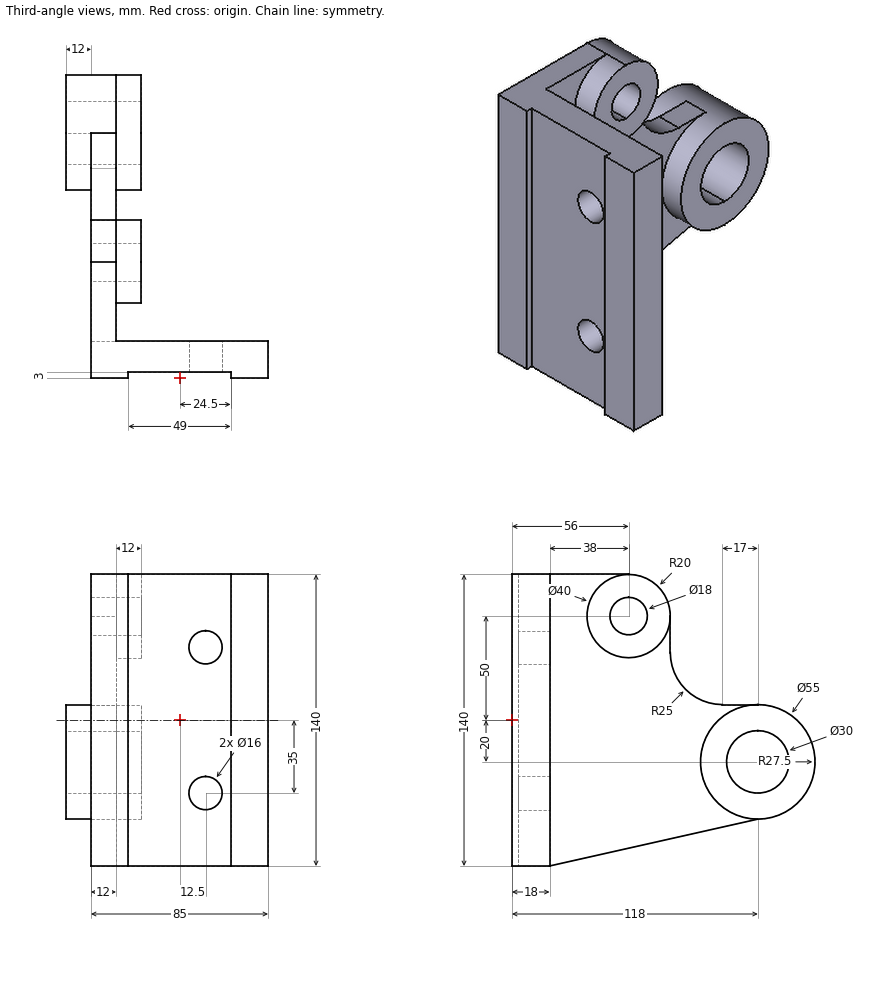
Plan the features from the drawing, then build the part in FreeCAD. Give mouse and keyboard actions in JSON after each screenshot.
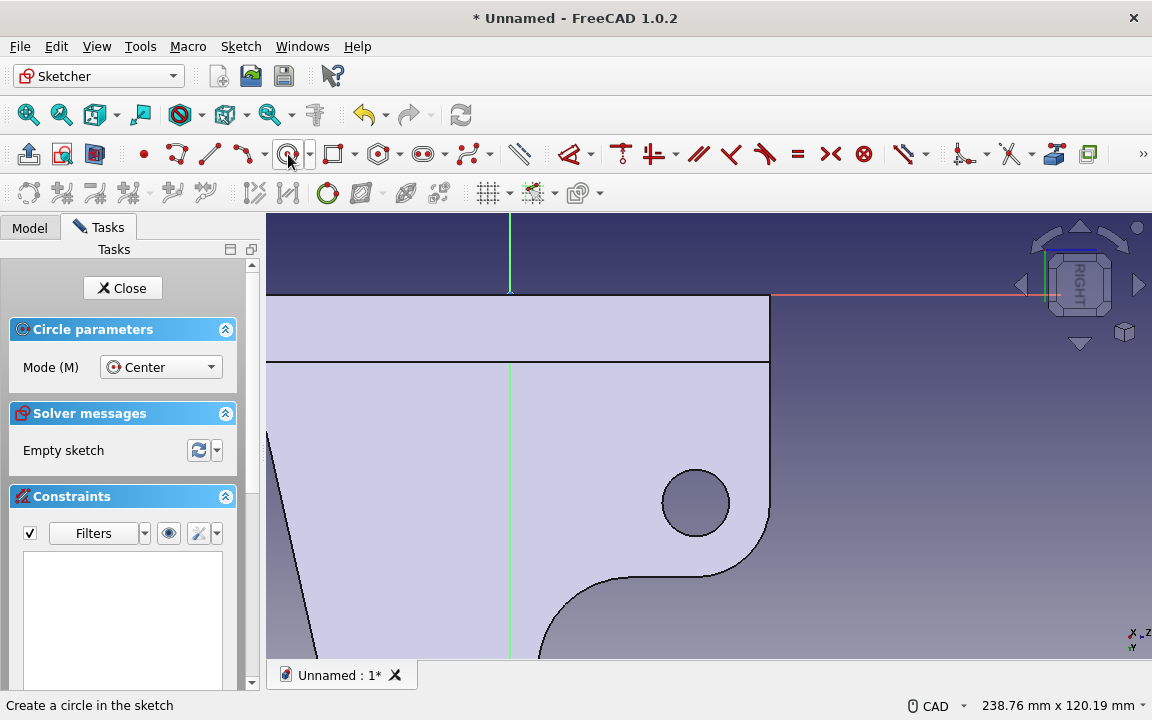
{"action": "left_click", "coordinate": [696, 503]}
{"action": "mouse_move", "coordinate": [748, 451]}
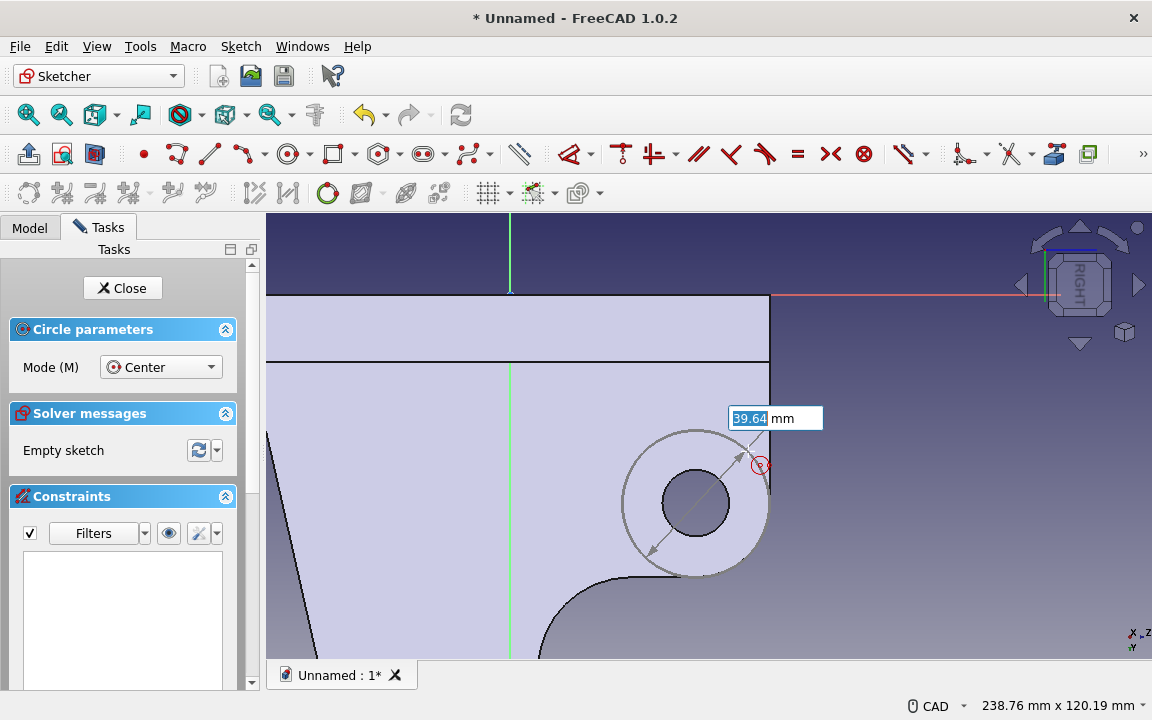
{"action": "type", "text": "40"}
{"action": "key", "text": "Return"}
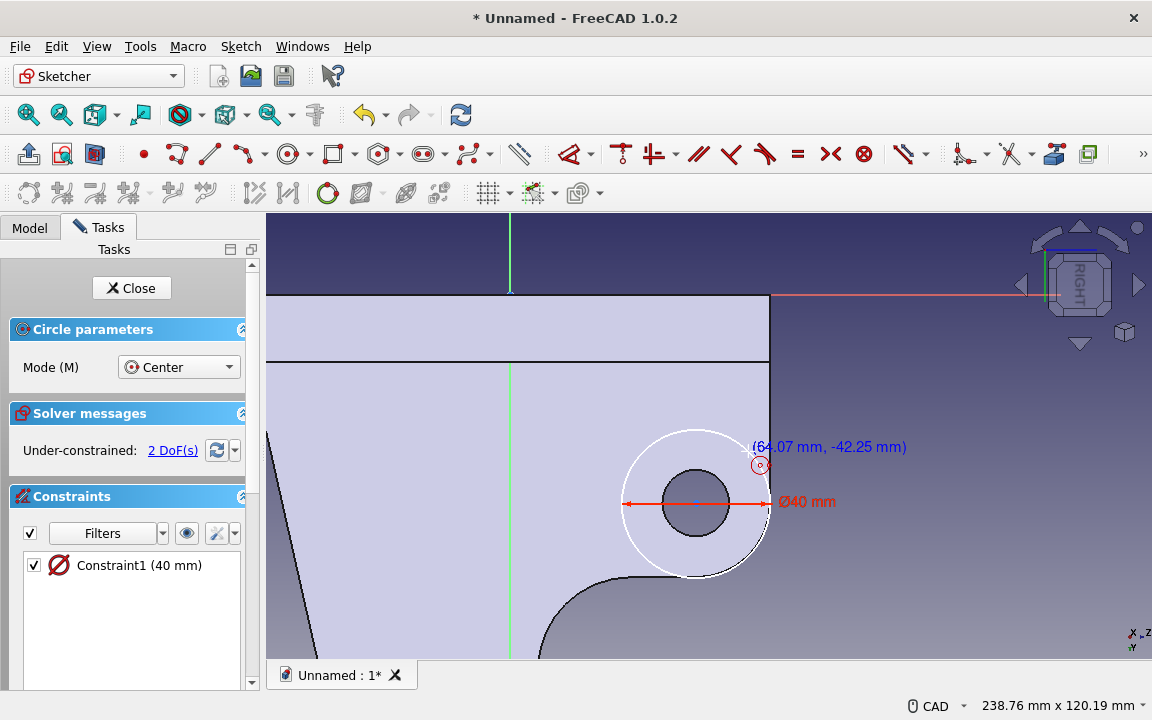
{"action": "left_click", "coordinate": [696, 504]}
{"action": "mouse_move", "coordinate": [719, 479]}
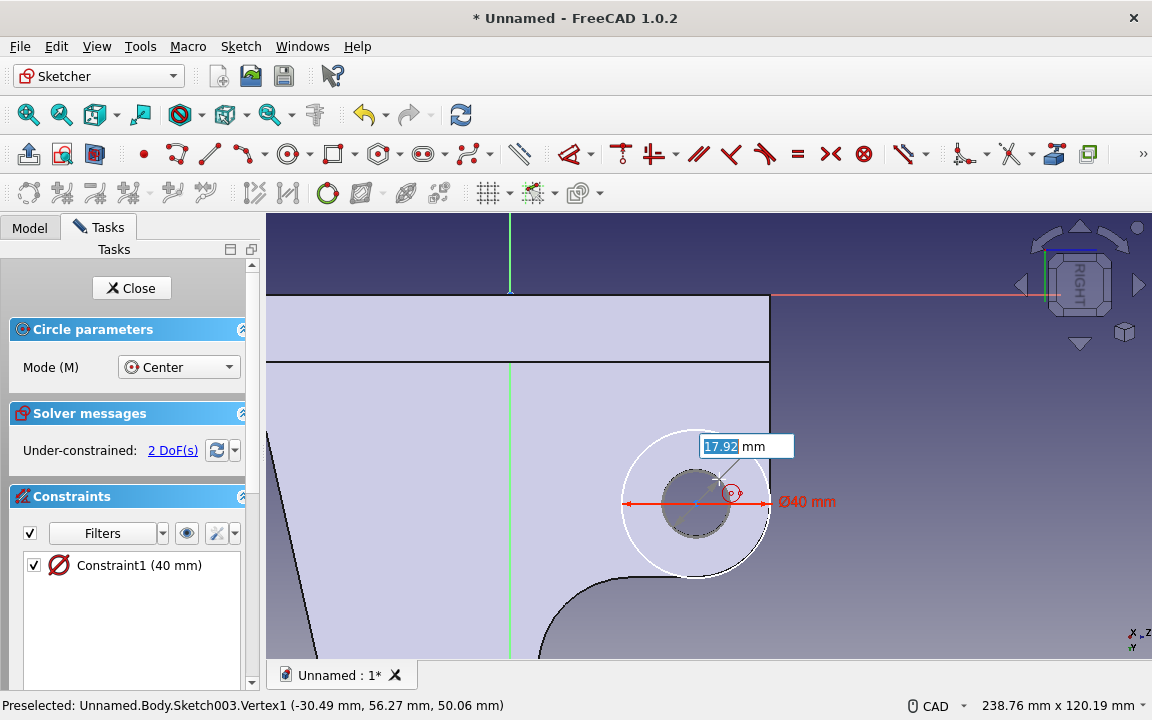
{"action": "type", "text": "18"}
{"action": "key", "text": "Return"}
{"action": "key", "text": "Escape"}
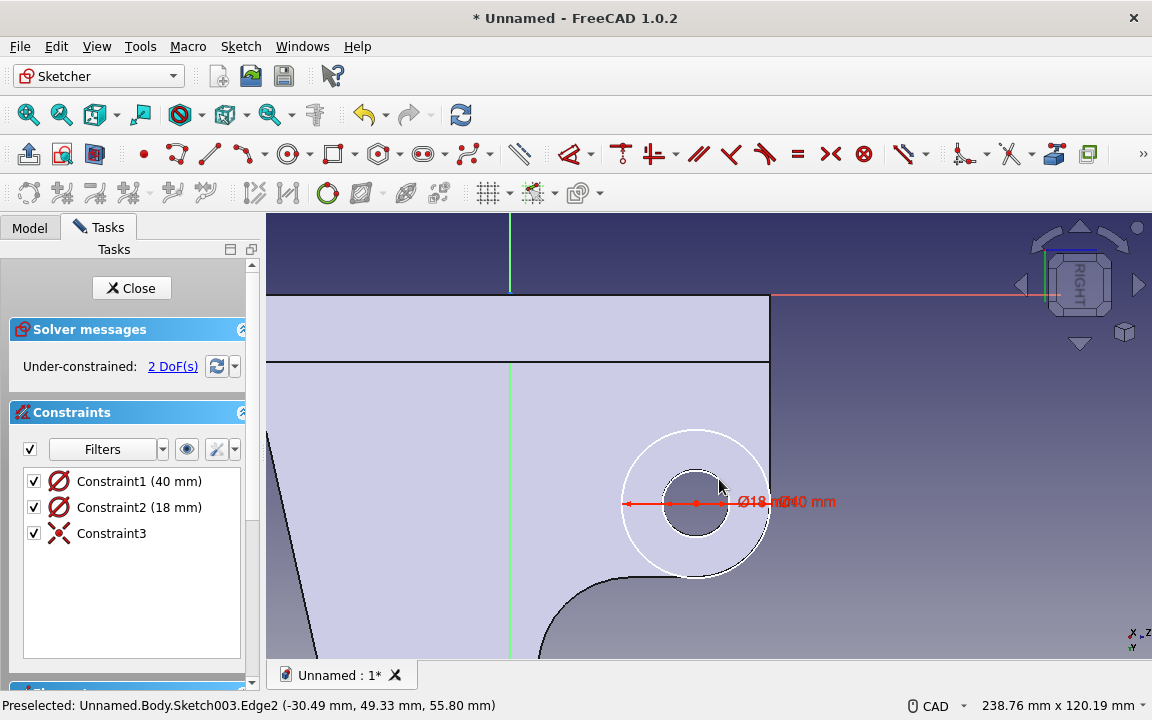
{"action": "left_click", "coordinate": [568, 154]}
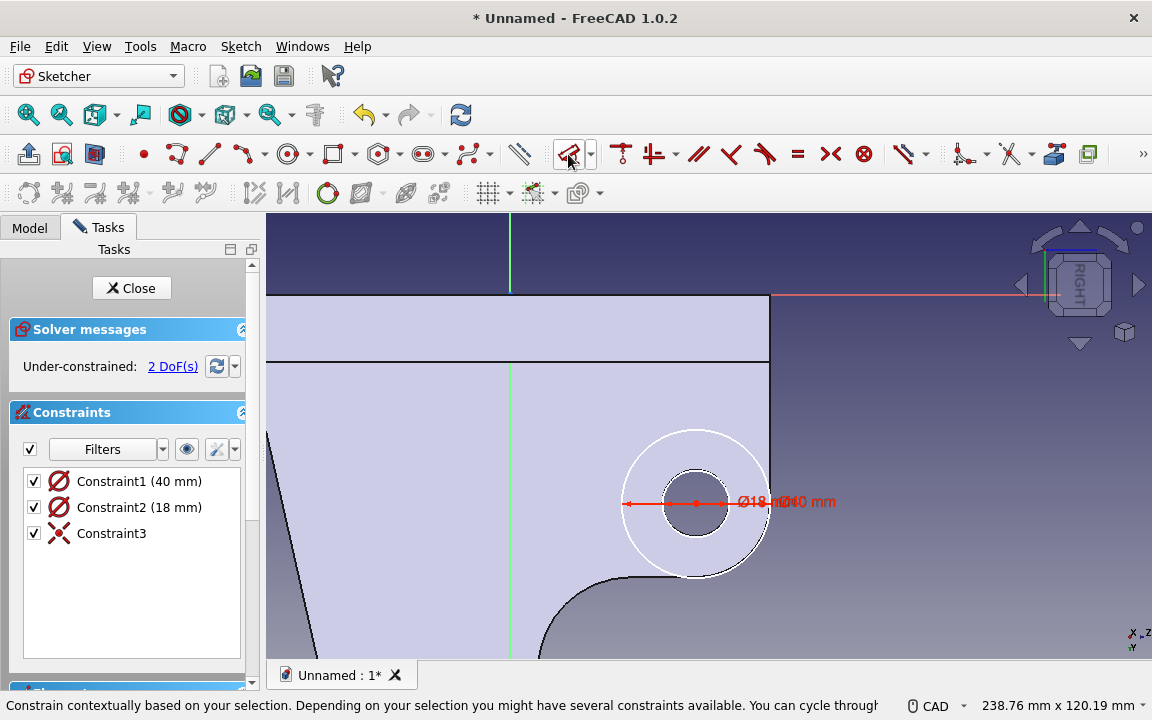
{"action": "left_click", "coordinate": [696, 504]}
{"action": "left_click", "coordinate": [603, 261]}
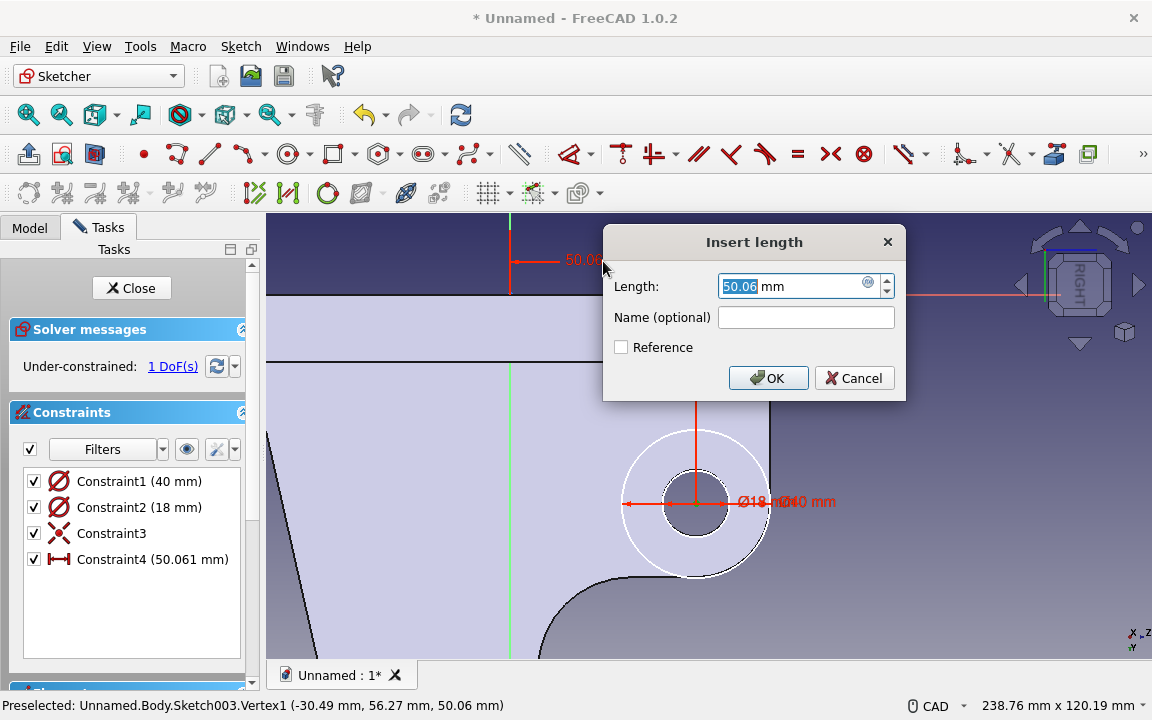
{"action": "type", "text": "50"}
{"action": "key", "text": "Return"}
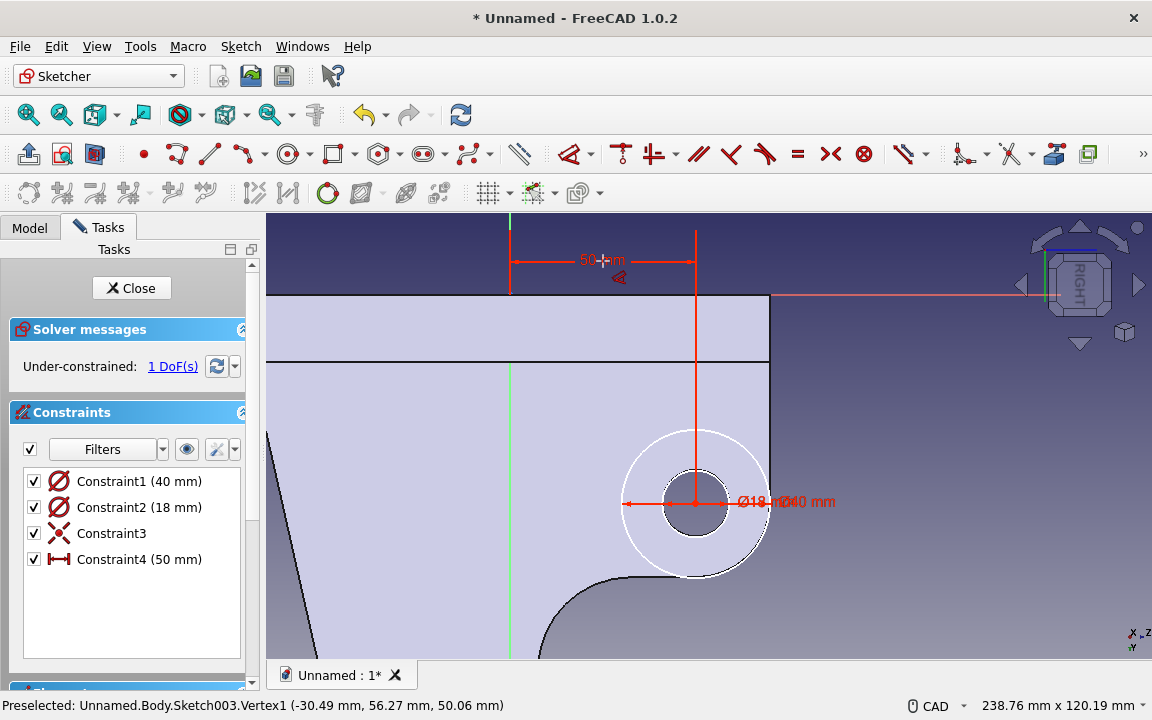
{"action": "left_click", "coordinate": [696, 504]}
{"action": "left_click", "coordinate": [476, 400]}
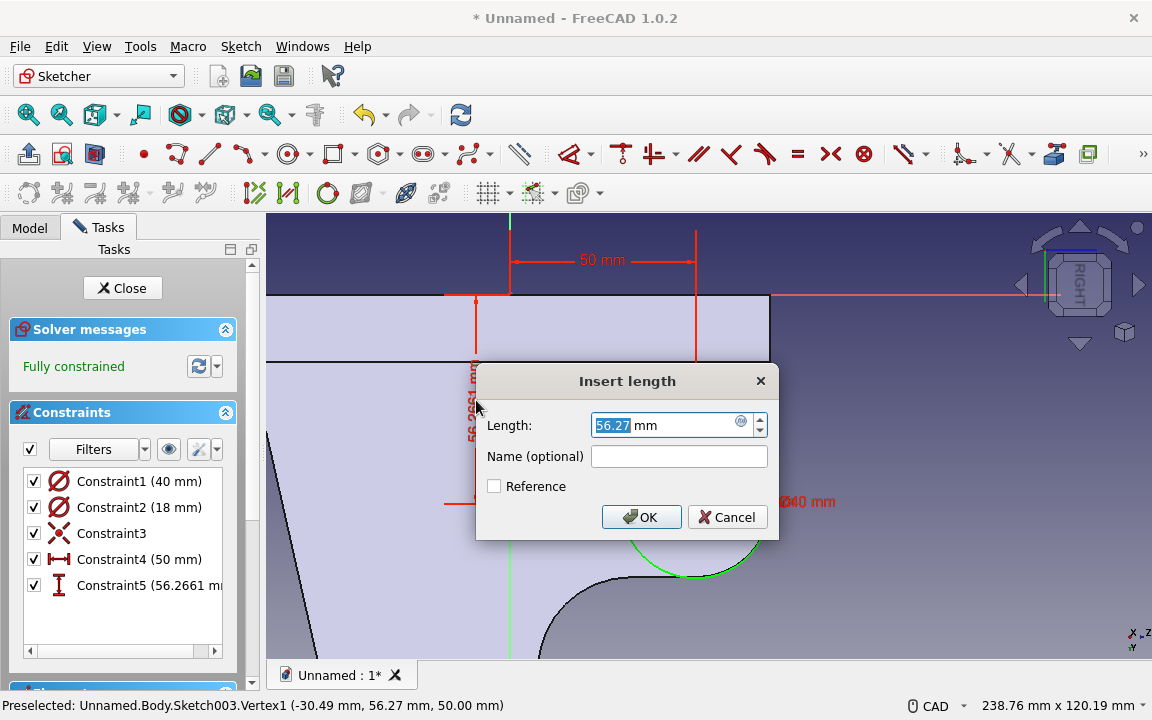
{"action": "type", "text": "56"}
{"action": "key", "text": "Return"}
{"action": "key", "text": "Escape"}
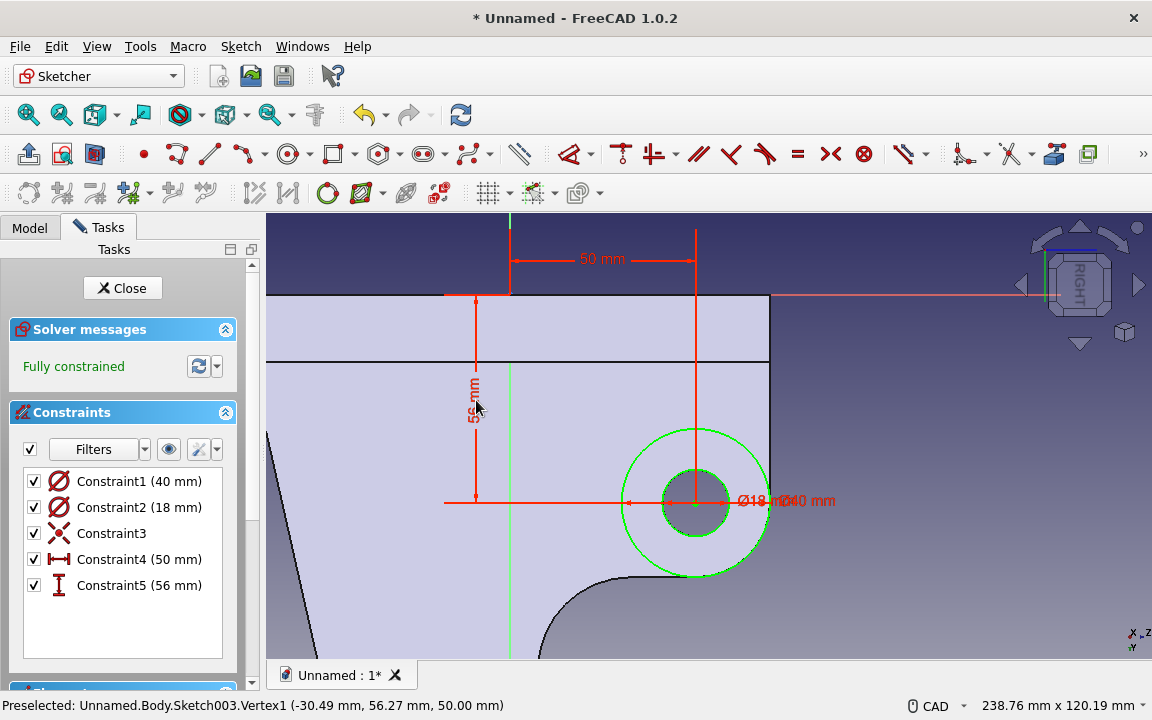
{"action": "left_click", "coordinate": [123, 288]}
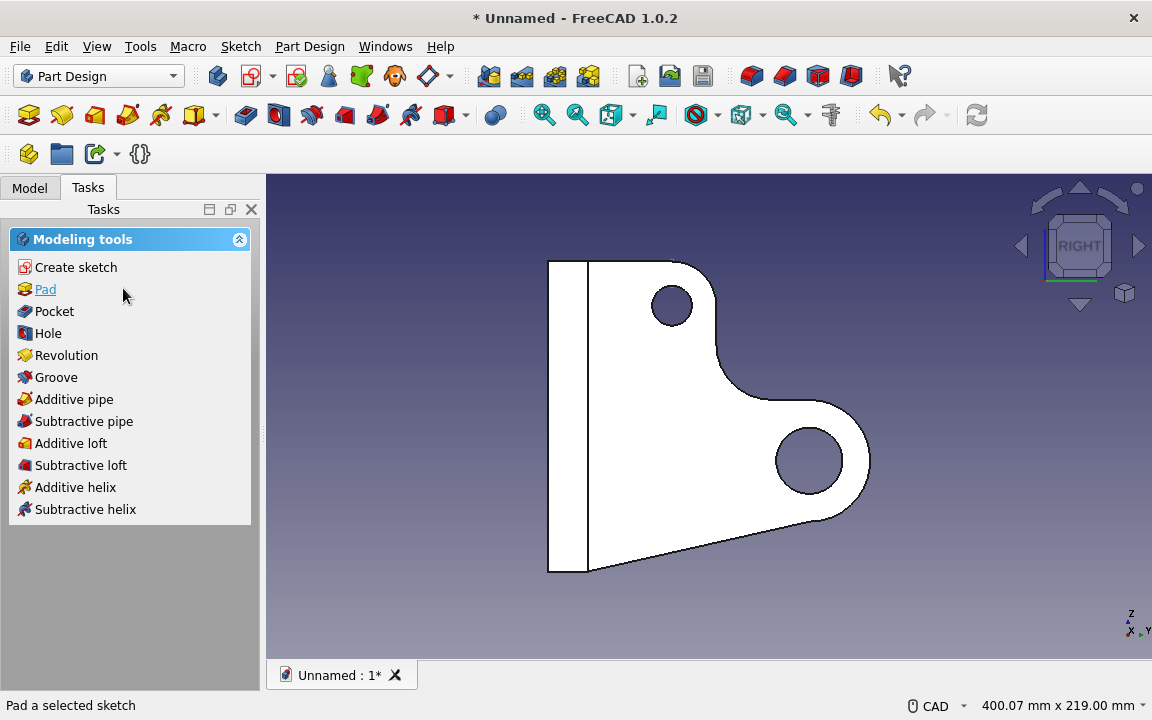
{"action": "left_click", "coordinate": [29, 116]}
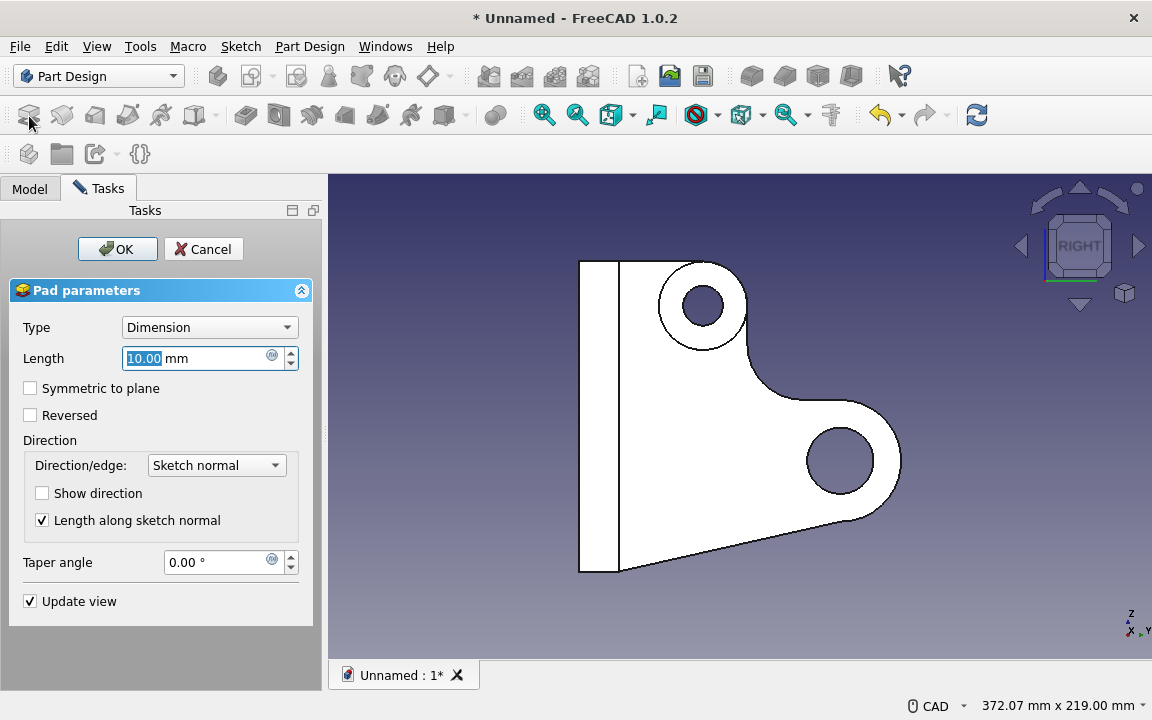
{"action": "type", "text": "12"}
{"action": "key", "text": "Tab"}